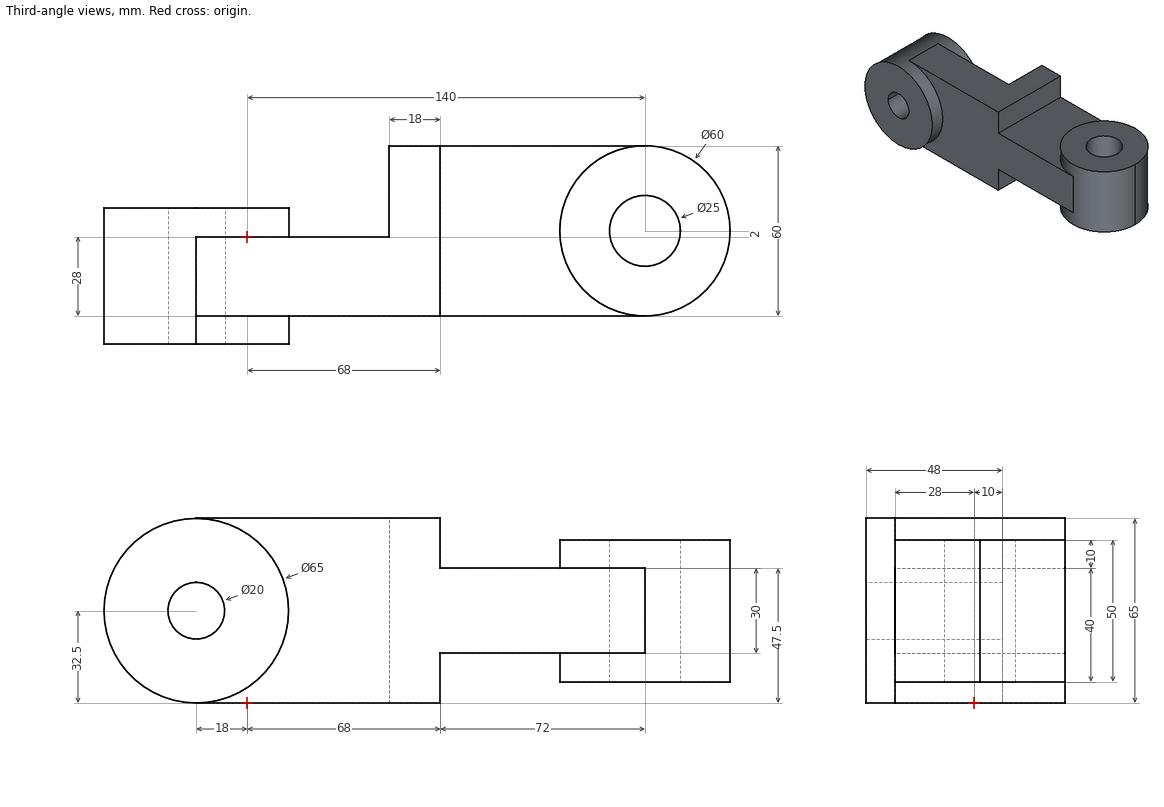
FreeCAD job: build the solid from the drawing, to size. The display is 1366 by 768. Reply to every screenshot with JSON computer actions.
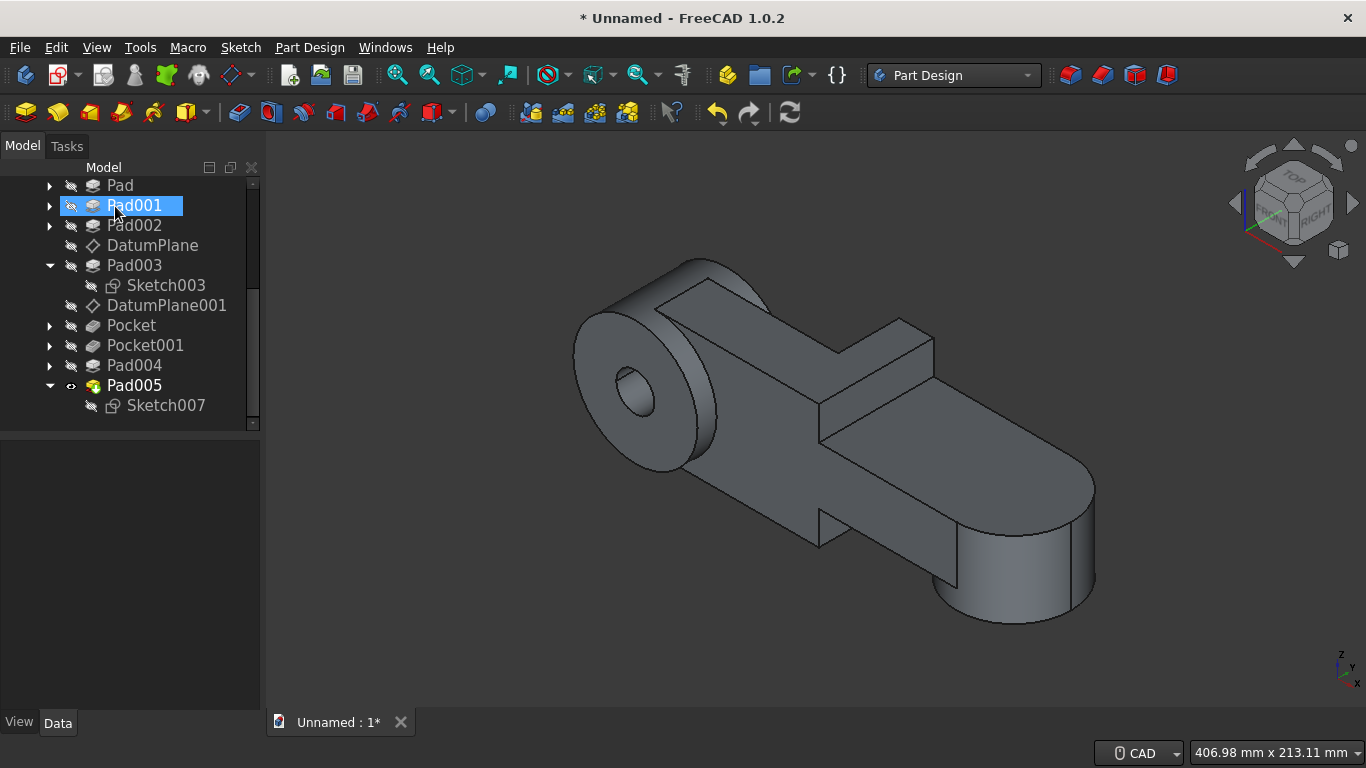
{"action": "scroll", "coordinate": [140, 301], "scroll_direction": "down", "scroll_amount": 3}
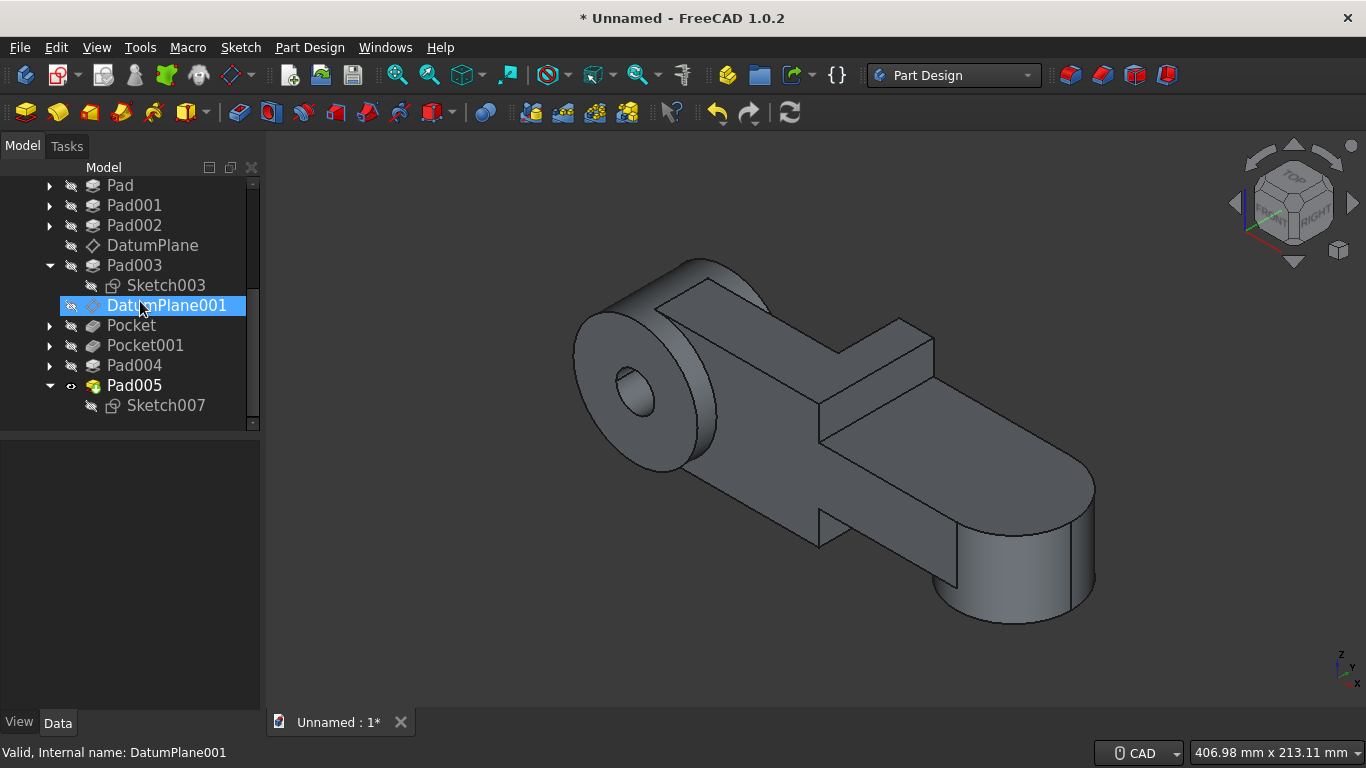
{"action": "scroll", "coordinate": [140, 301], "scroll_direction": "up", "scroll_amount": 15}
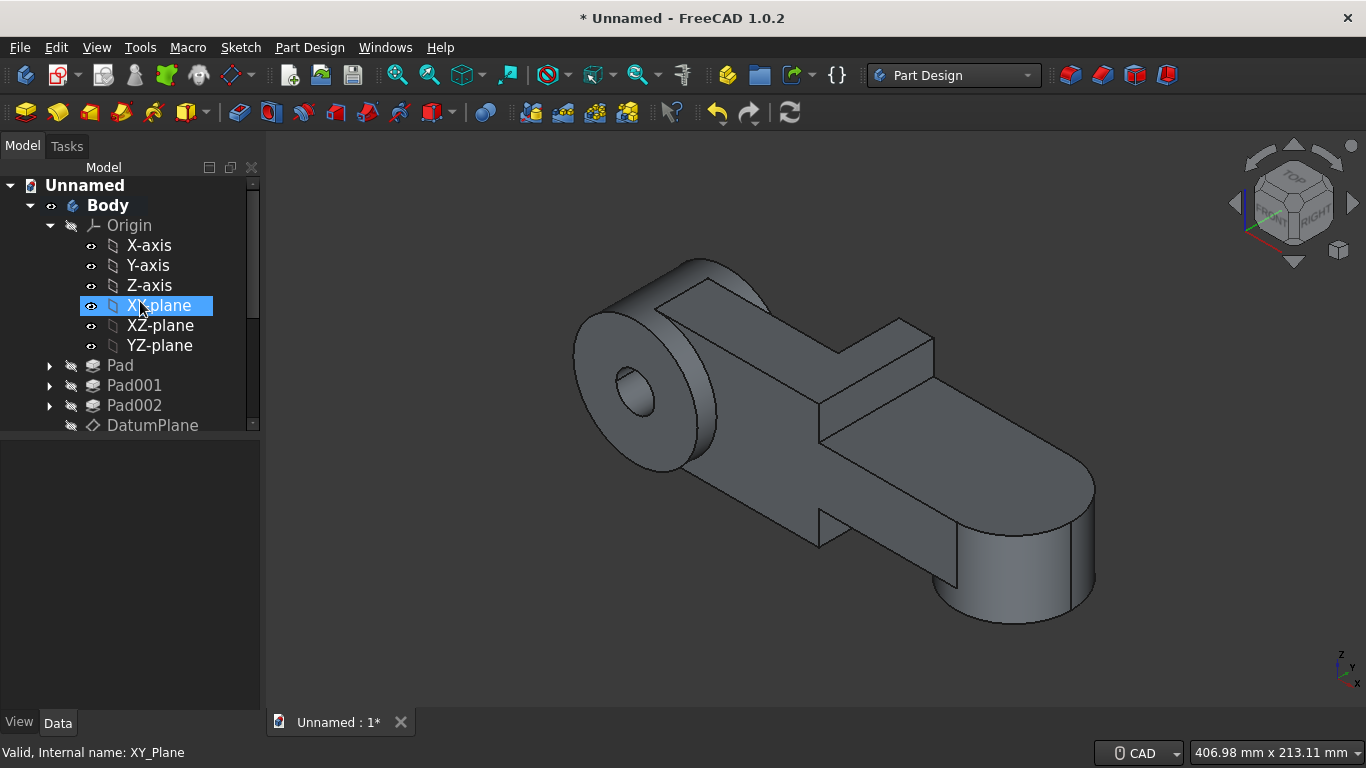
{"action": "left_click", "coordinate": [136, 306]}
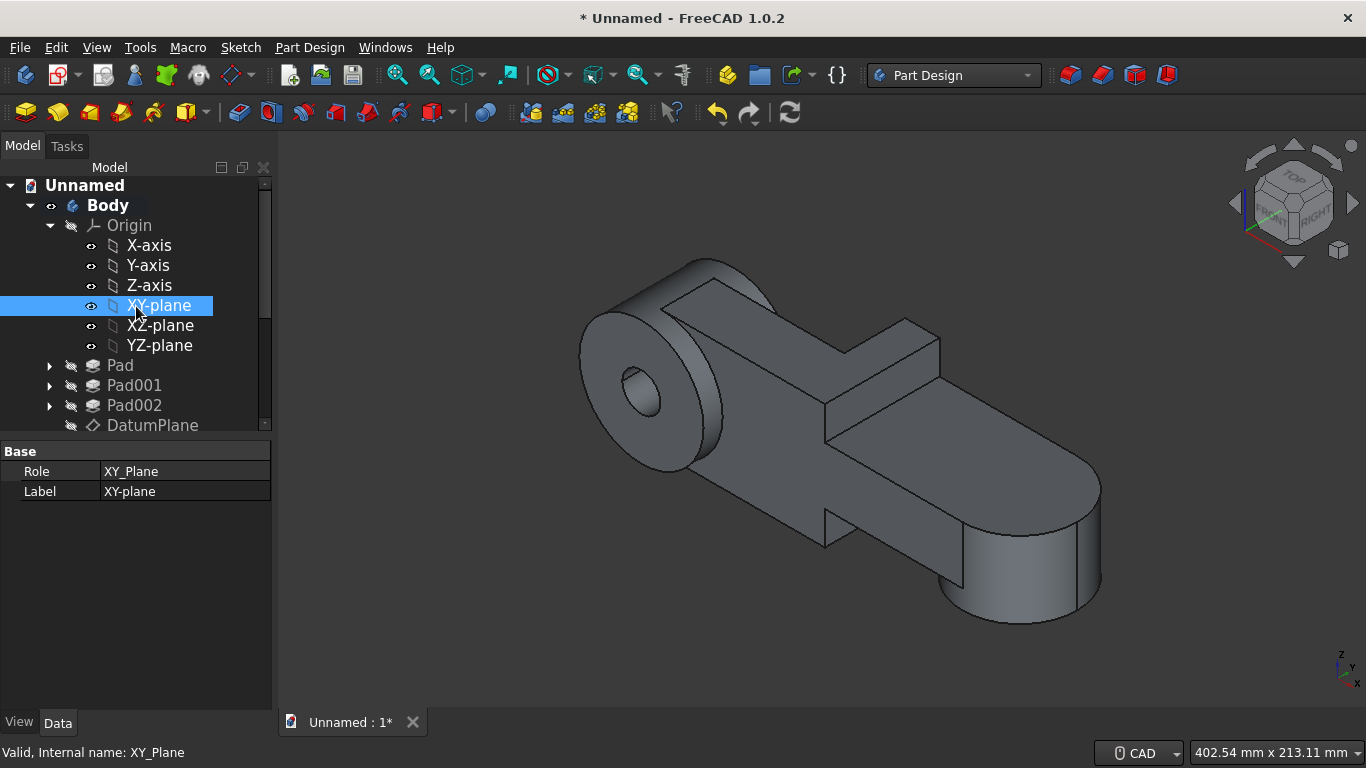
{"action": "left_click", "coordinate": [232, 76]}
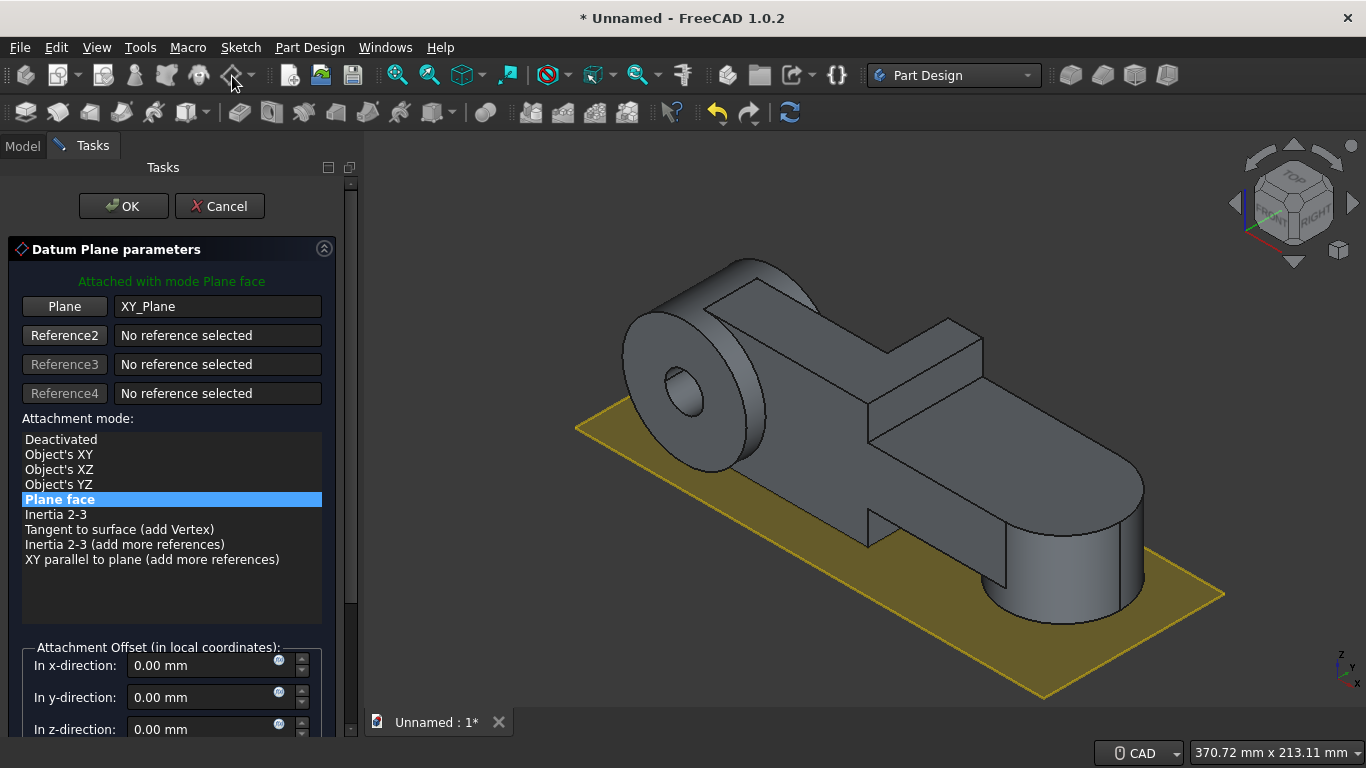
{"action": "scroll", "coordinate": [351, 456], "scroll_direction": "down", "scroll_amount": 2}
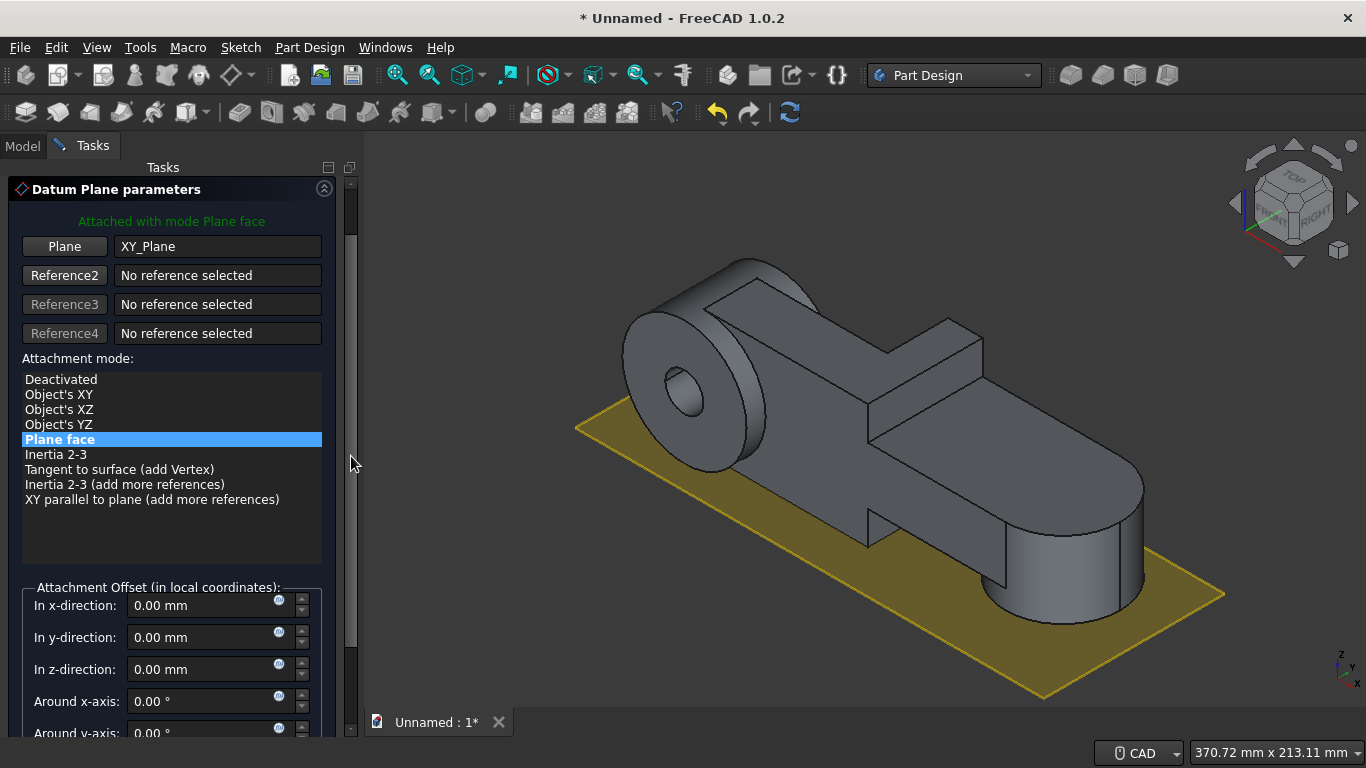
{"action": "triple_click", "coordinate": [210, 609]}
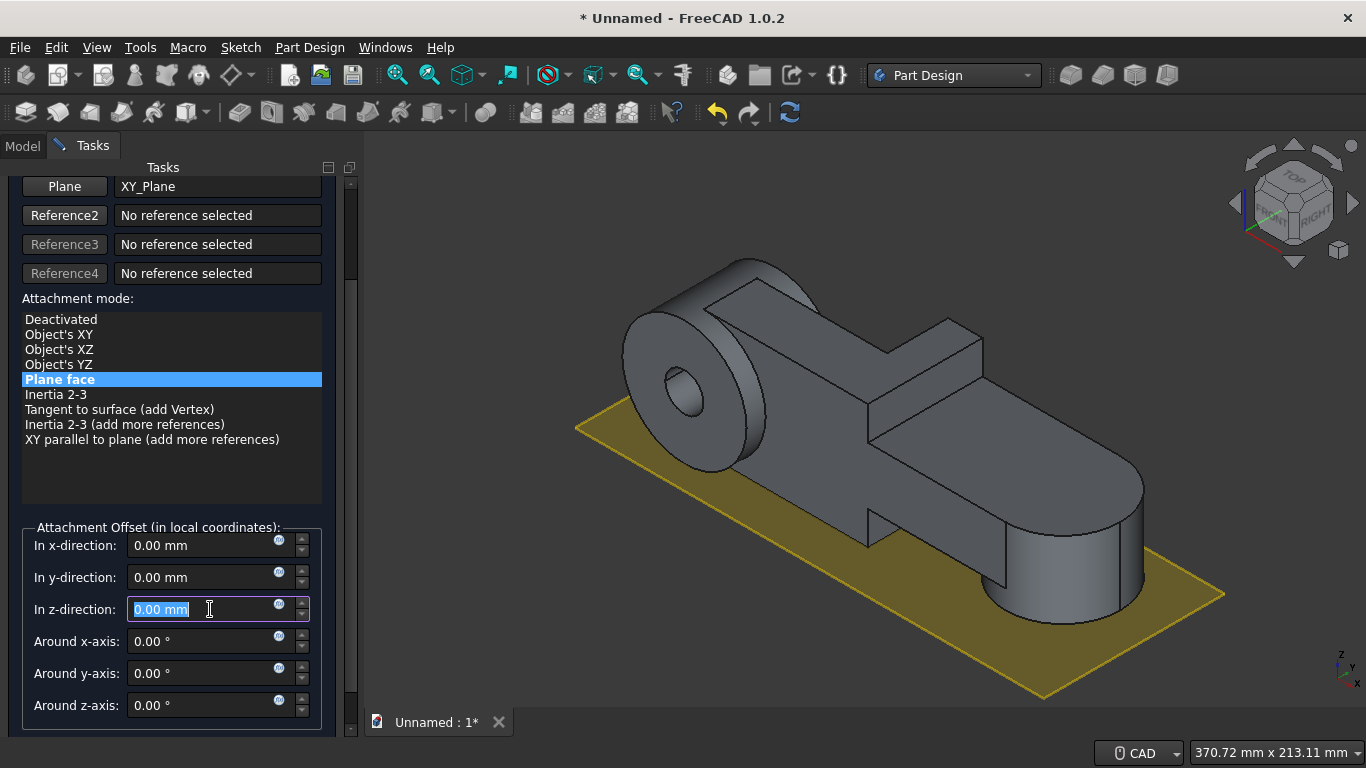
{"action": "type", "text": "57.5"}
{"action": "key", "text": "Tab"}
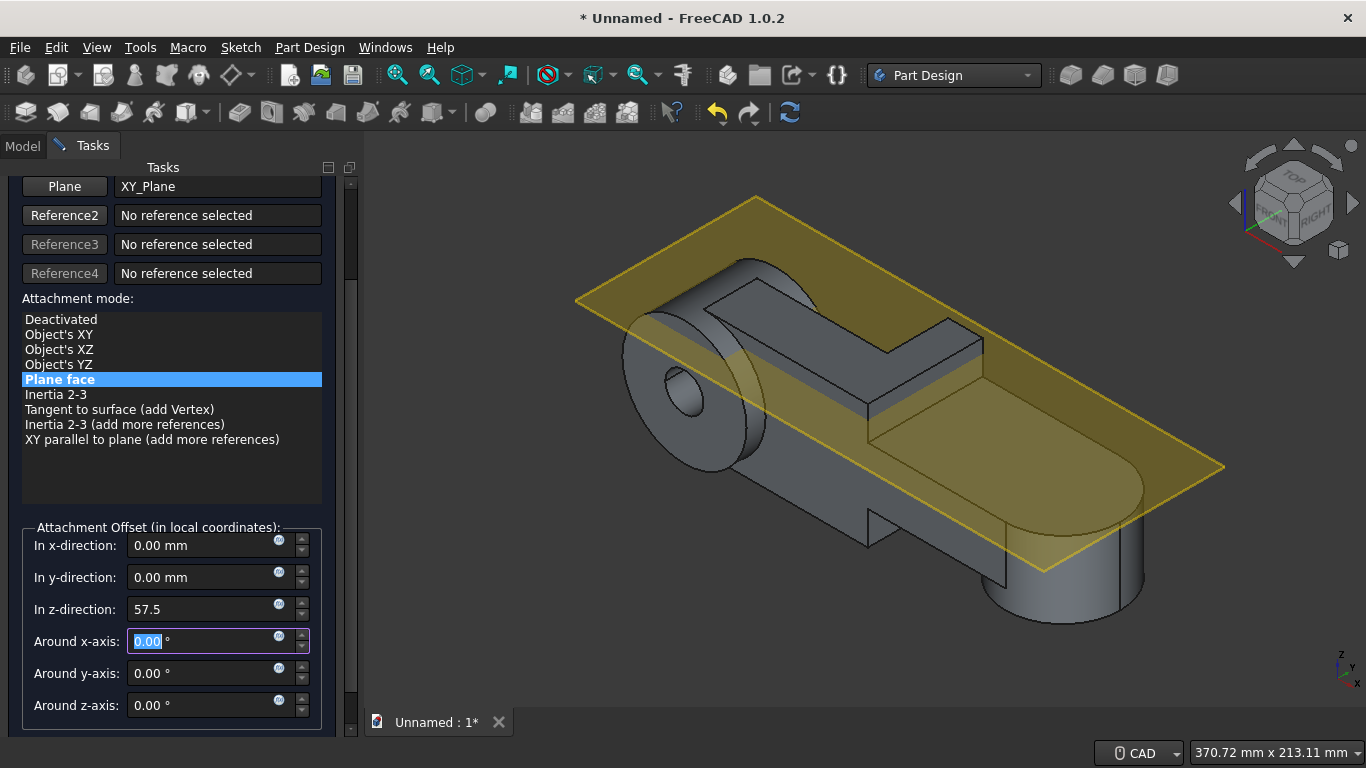
{"action": "scroll", "coordinate": [351, 456], "scroll_direction": "up", "scroll_amount": 3}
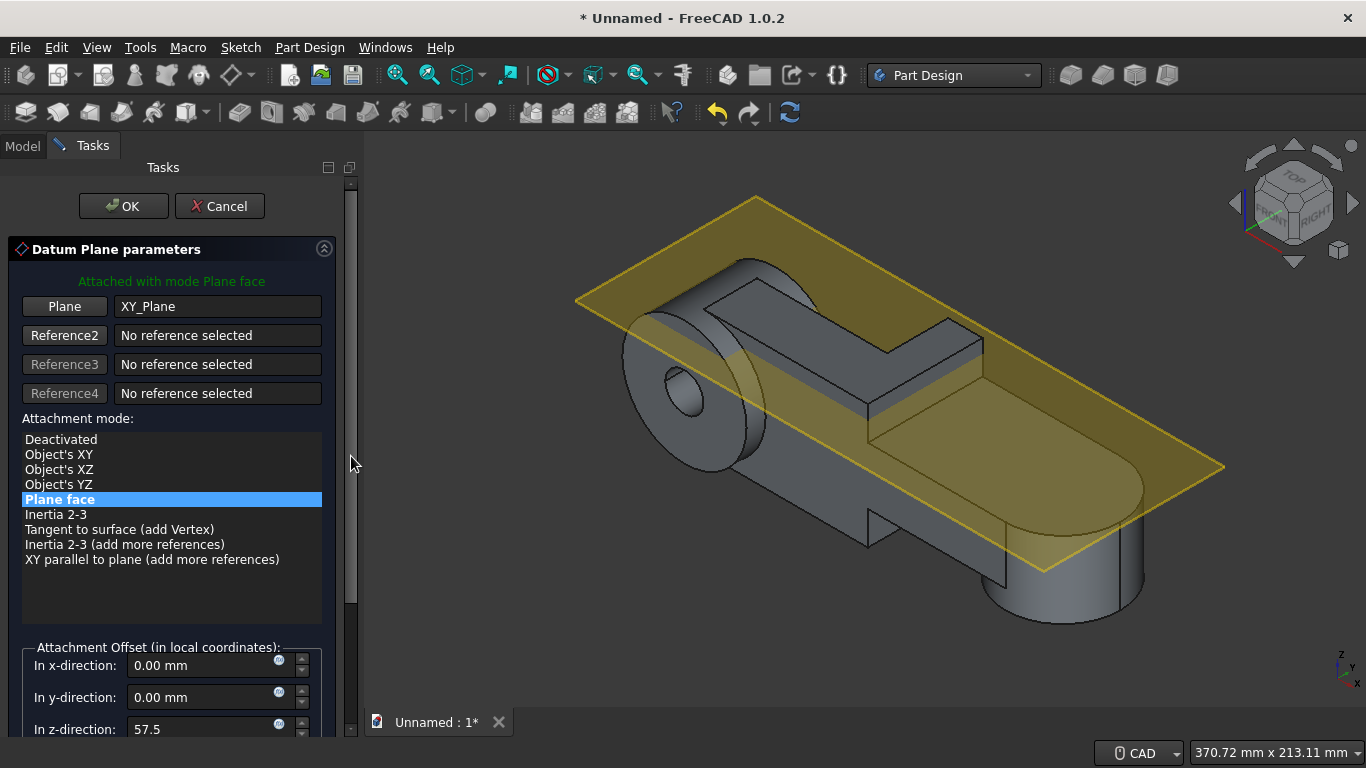
{"action": "left_click", "coordinate": [124, 206]}